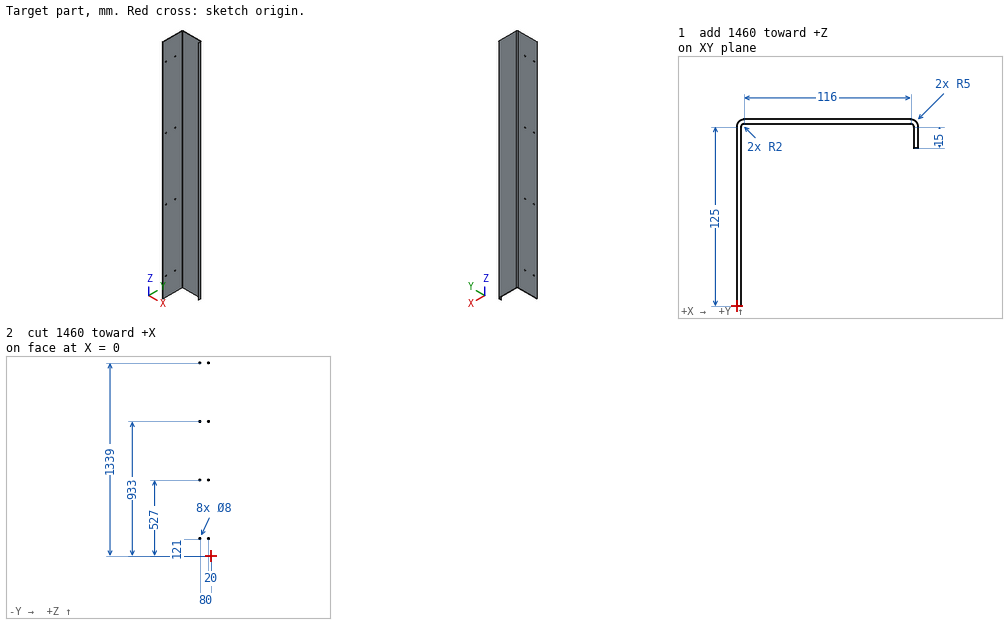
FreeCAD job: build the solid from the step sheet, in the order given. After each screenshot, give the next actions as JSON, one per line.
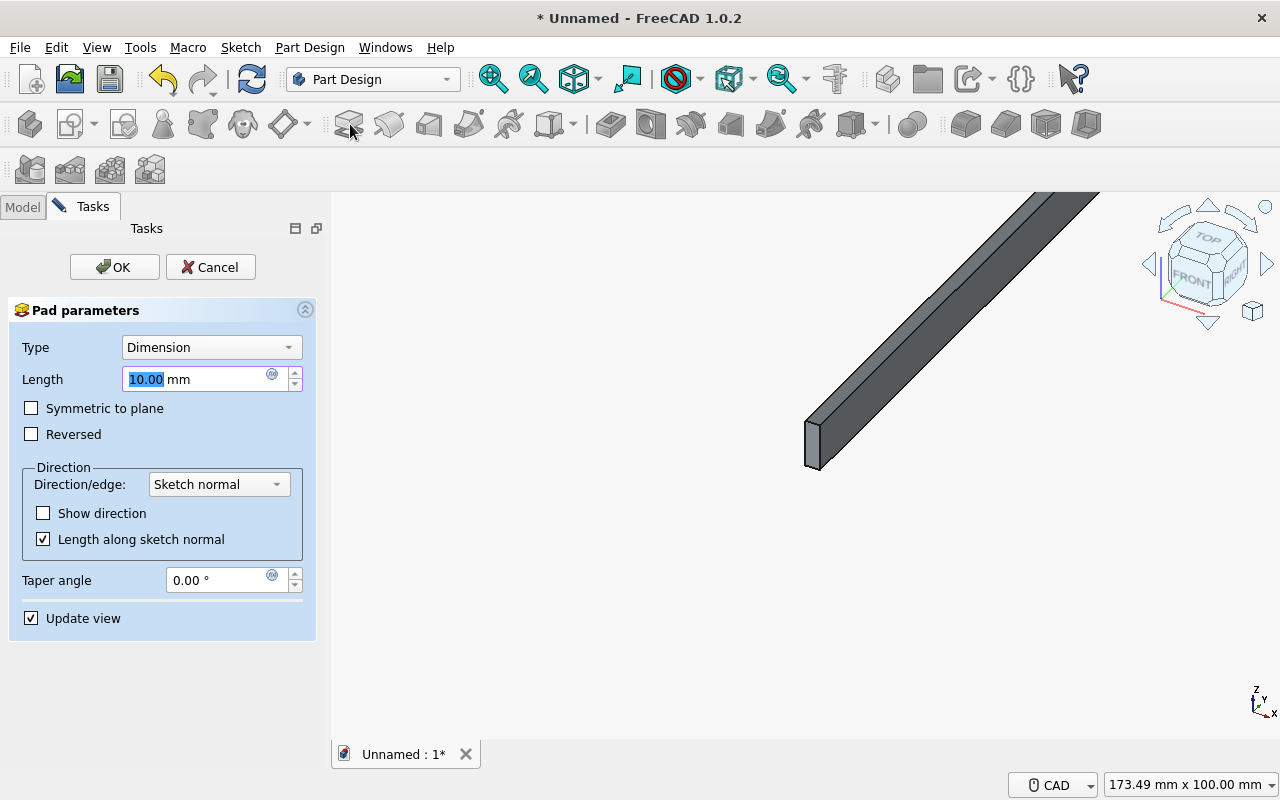
{"action": "type", "text": "1460"}
{"action": "key", "text": "Tab"}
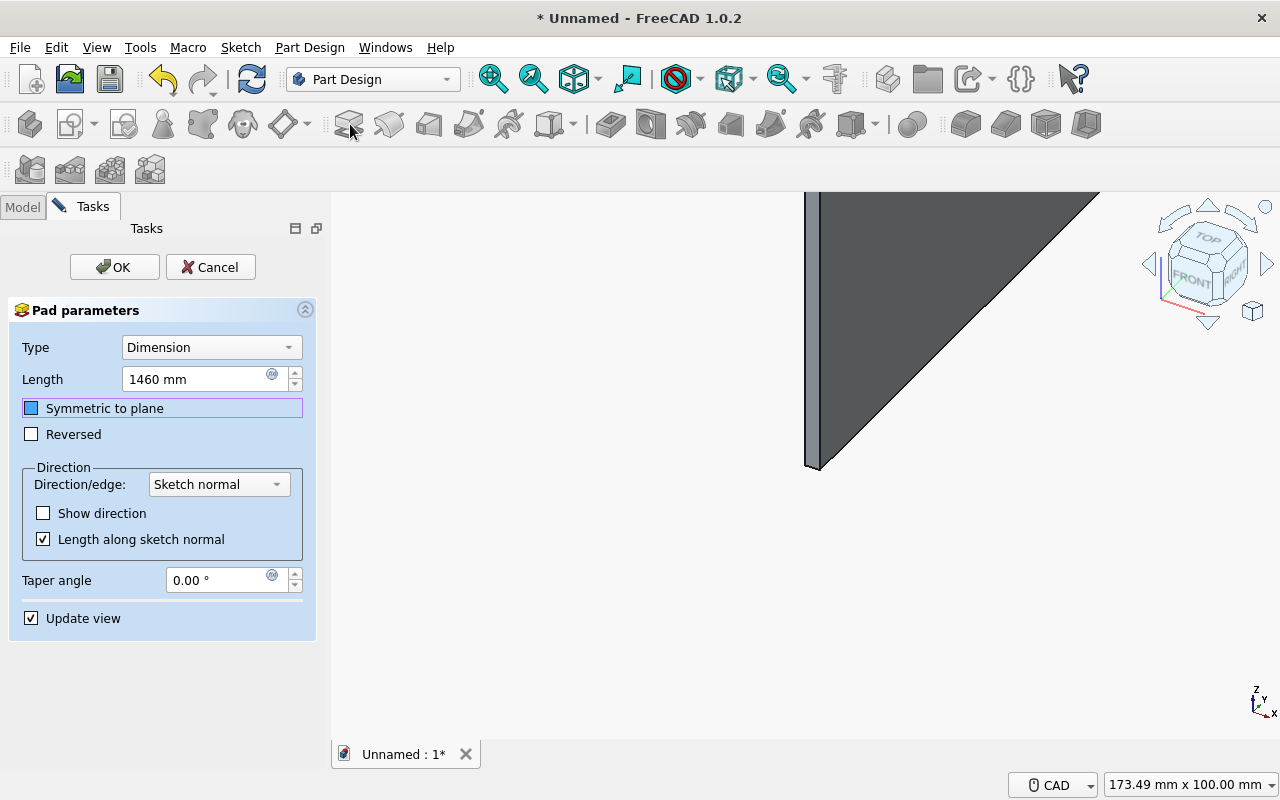
{"action": "left_click", "coordinate": [115, 267]}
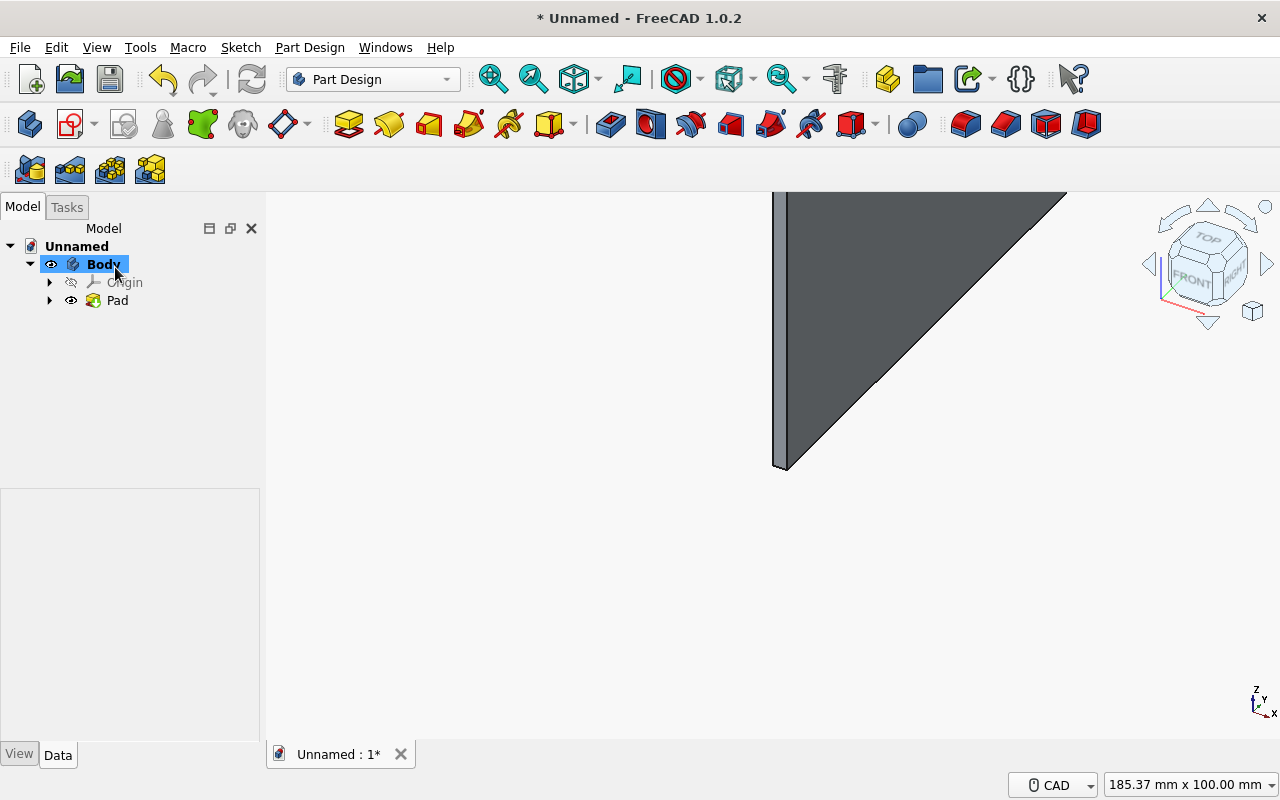
{"action": "key", "text": "v f"}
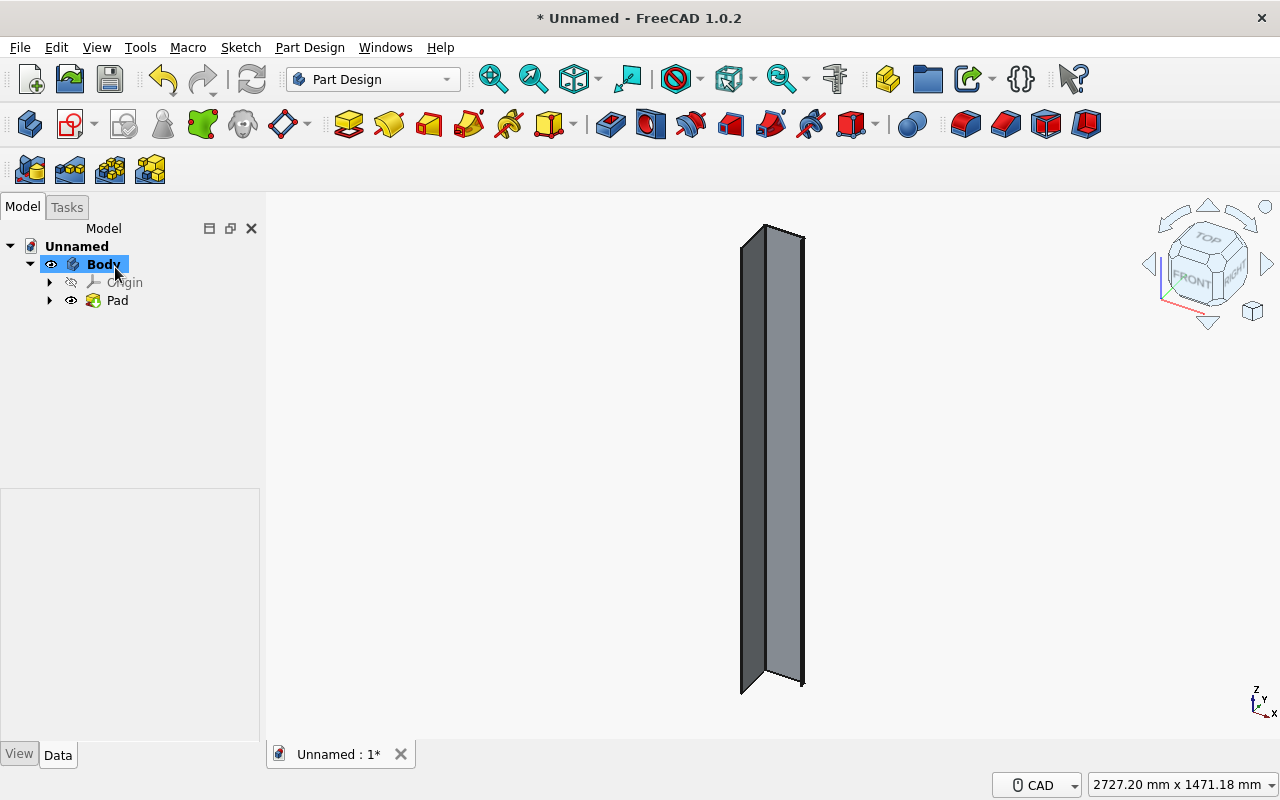
{"action": "key", "text": "6"}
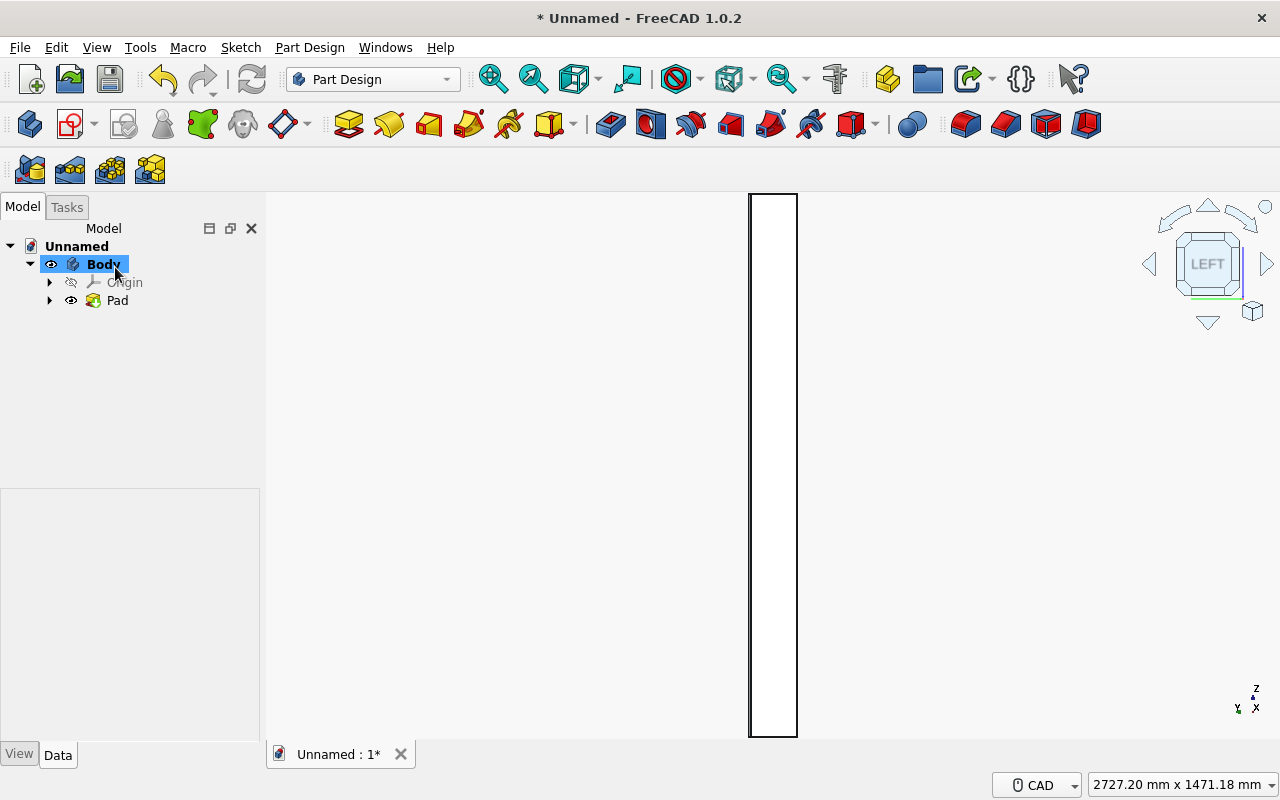
{"action": "left_click", "coordinate": [774, 232]}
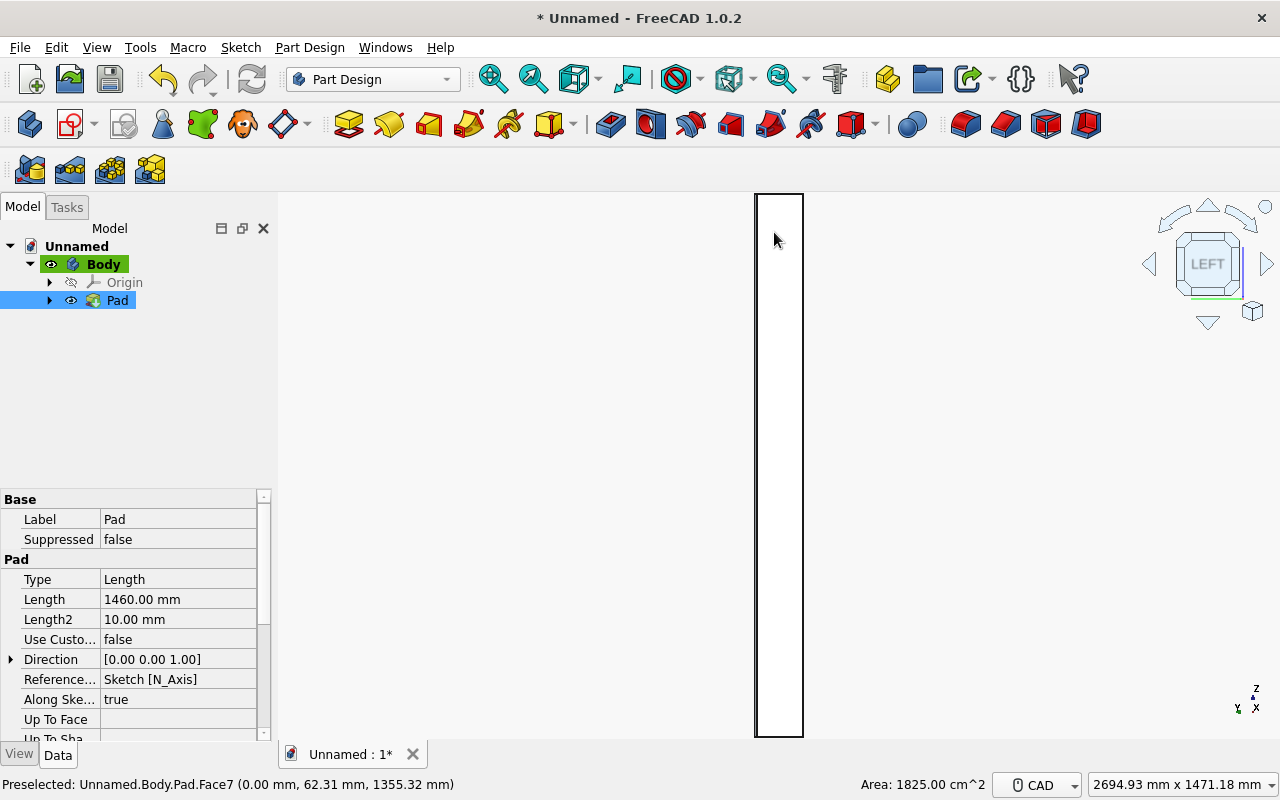
{"action": "left_click", "coordinate": [70, 124]}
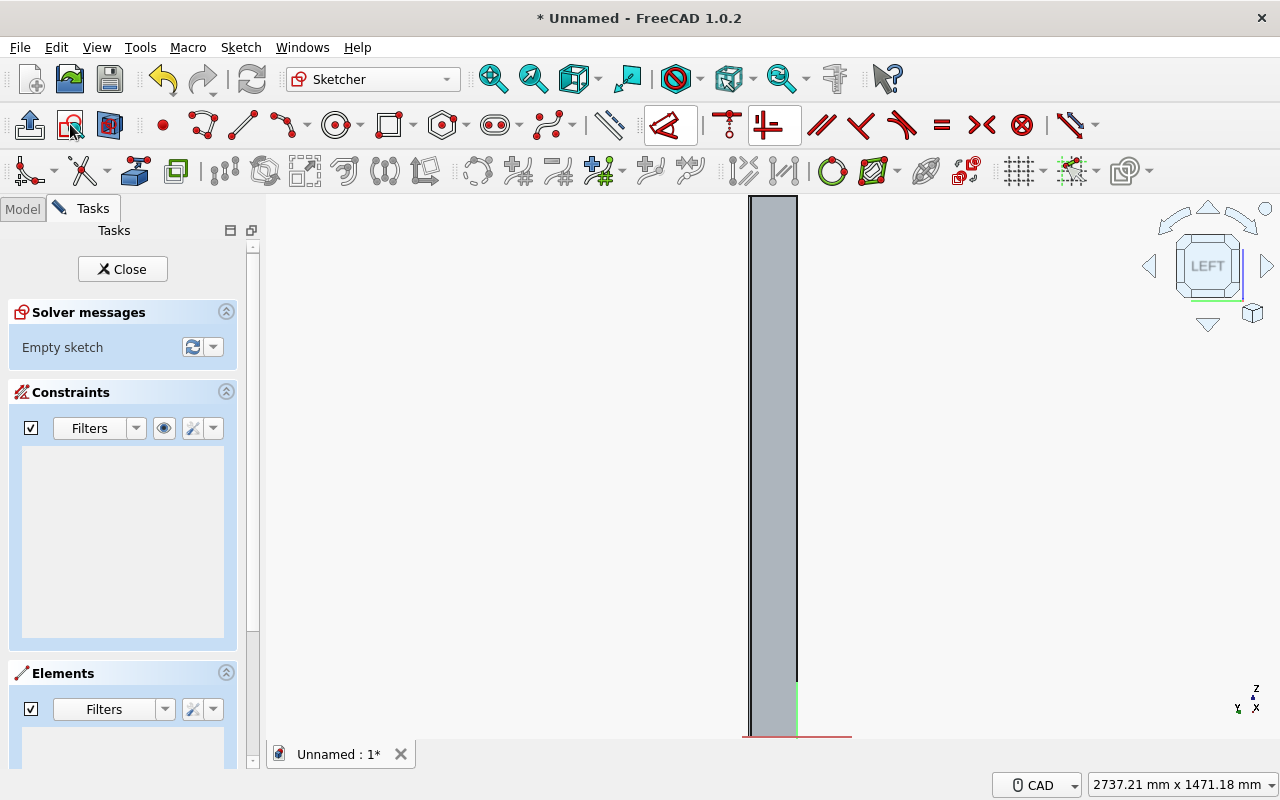
{"action": "scroll", "coordinate": [548, 422], "scroll_direction": "down", "scroll_amount": 2}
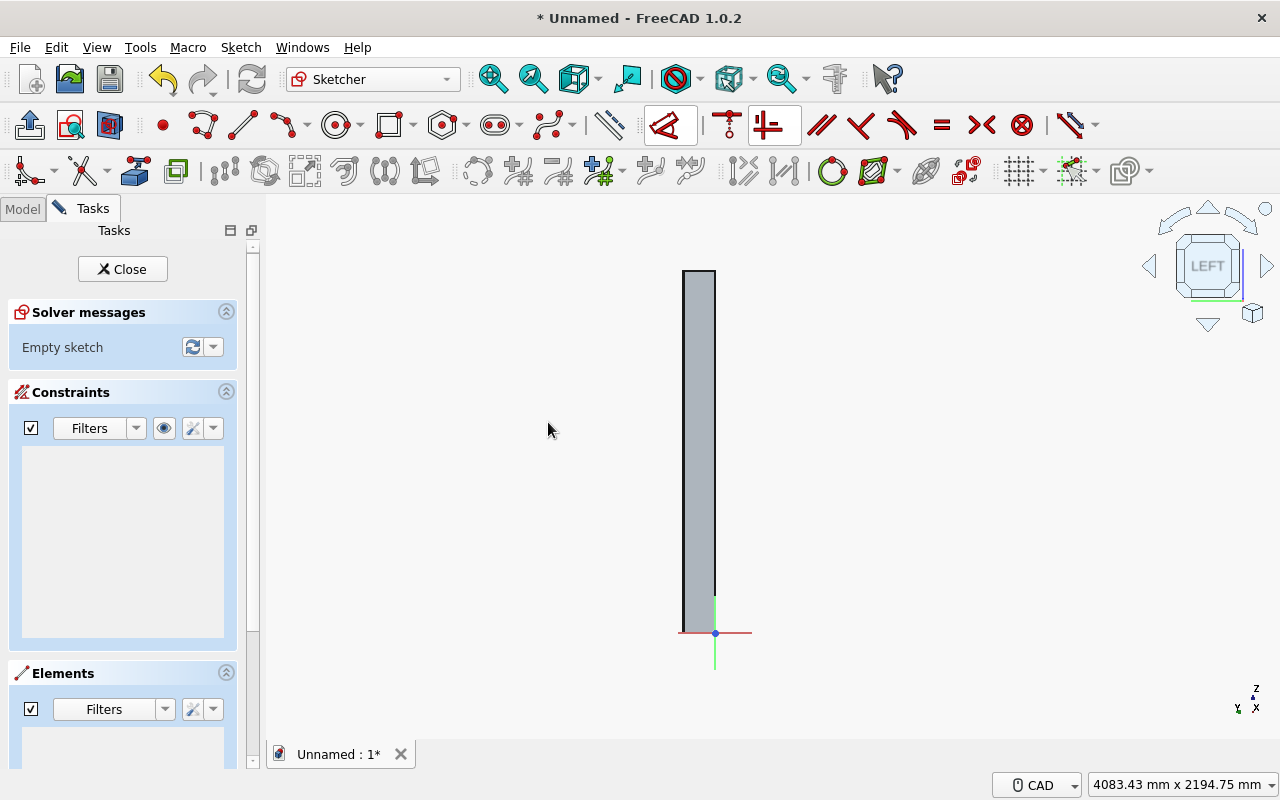
{"action": "left_click", "coordinate": [336, 126]}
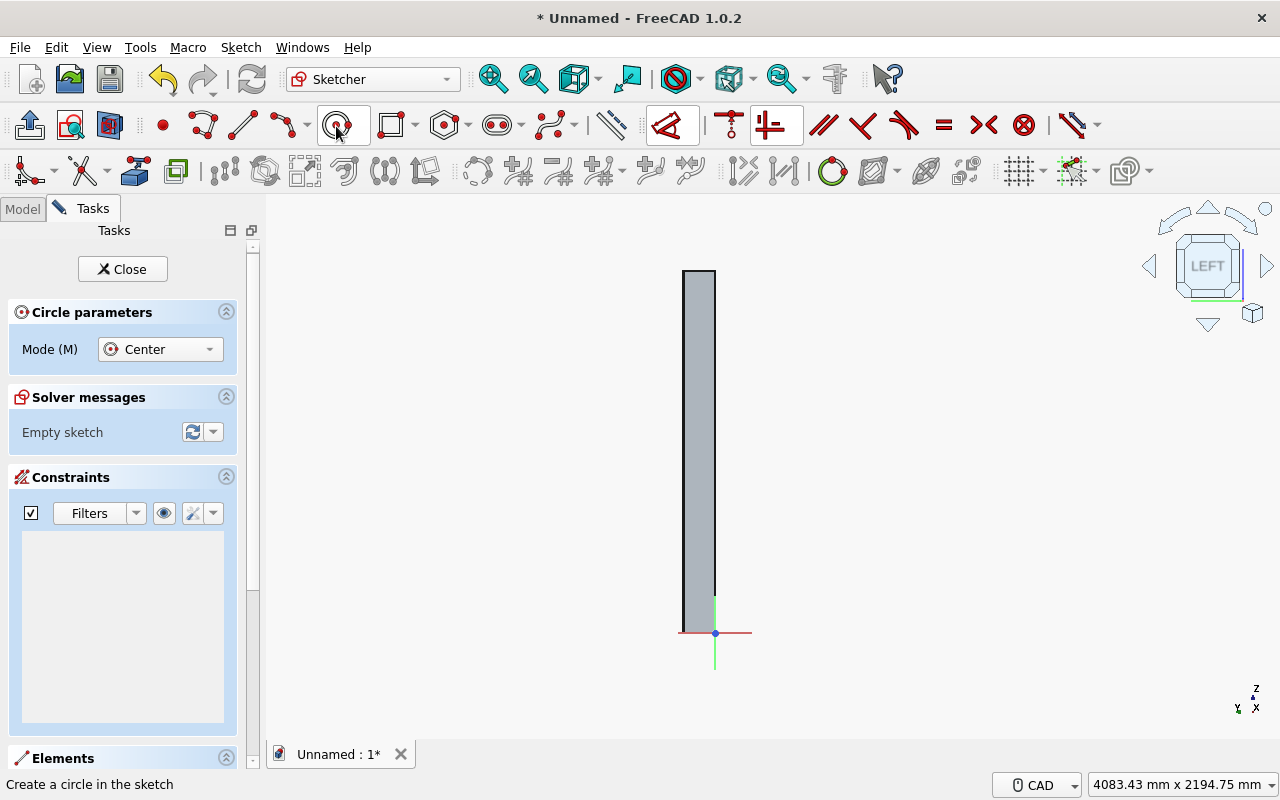
{"action": "scroll", "coordinate": [695, 603], "scroll_direction": "up", "scroll_amount": 16}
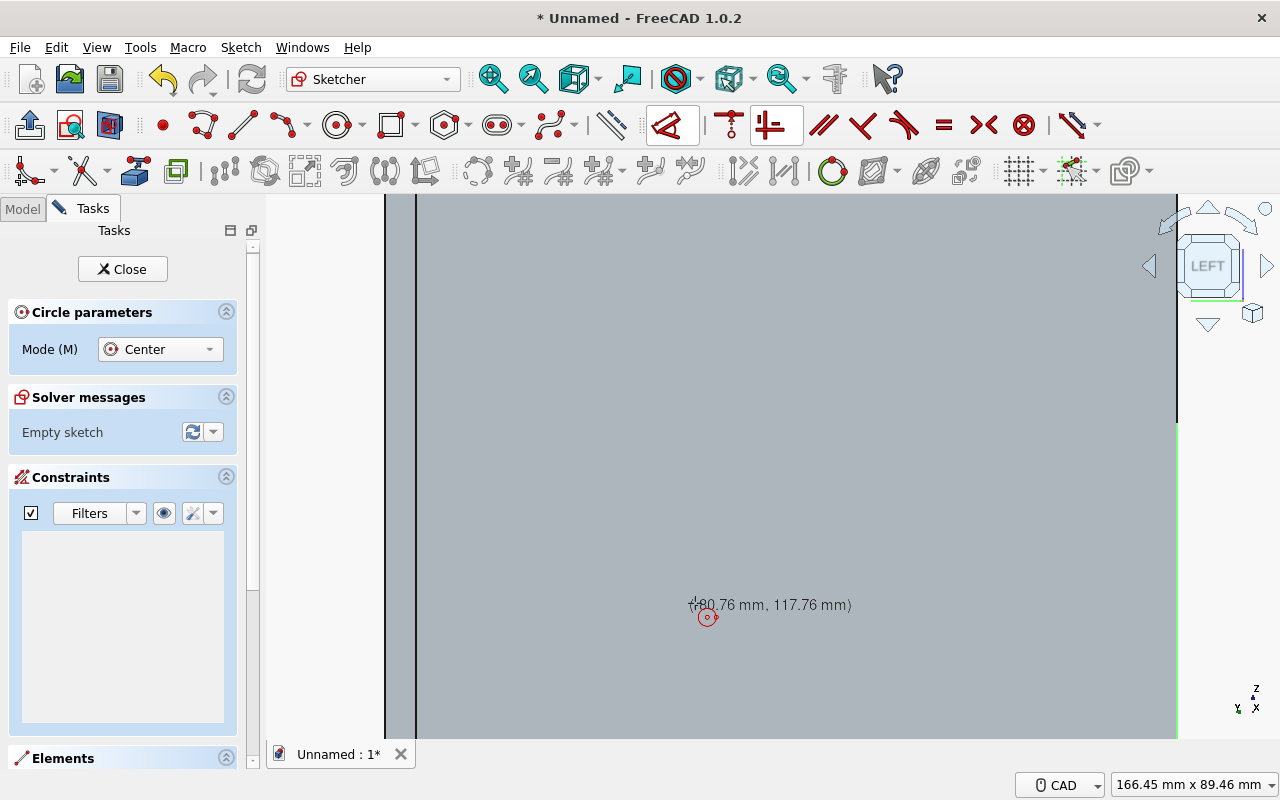
{"action": "scroll", "coordinate": [693, 636], "scroll_direction": "down", "scroll_amount": 15}